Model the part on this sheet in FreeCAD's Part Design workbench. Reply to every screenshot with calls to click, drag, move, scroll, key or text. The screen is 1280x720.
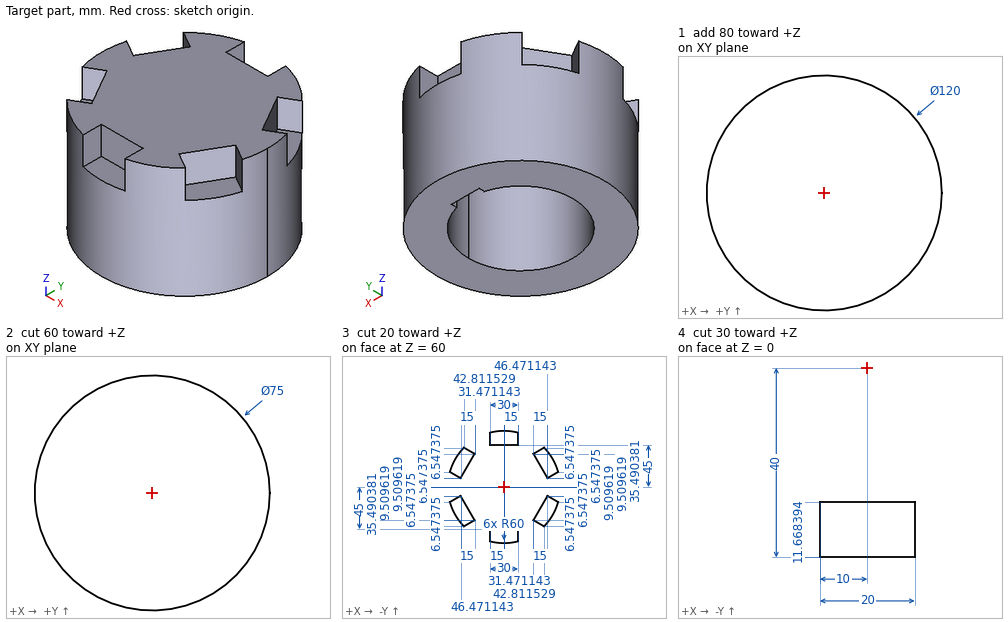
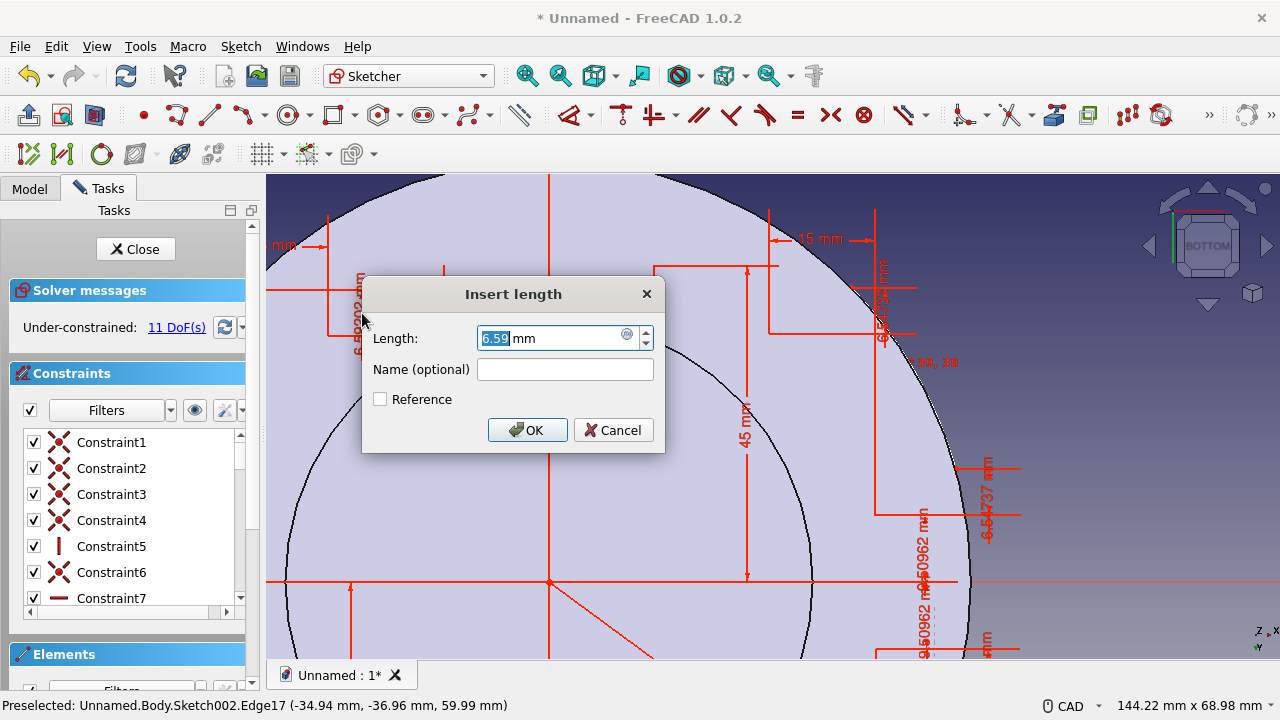
text(6.547375)
key(Return)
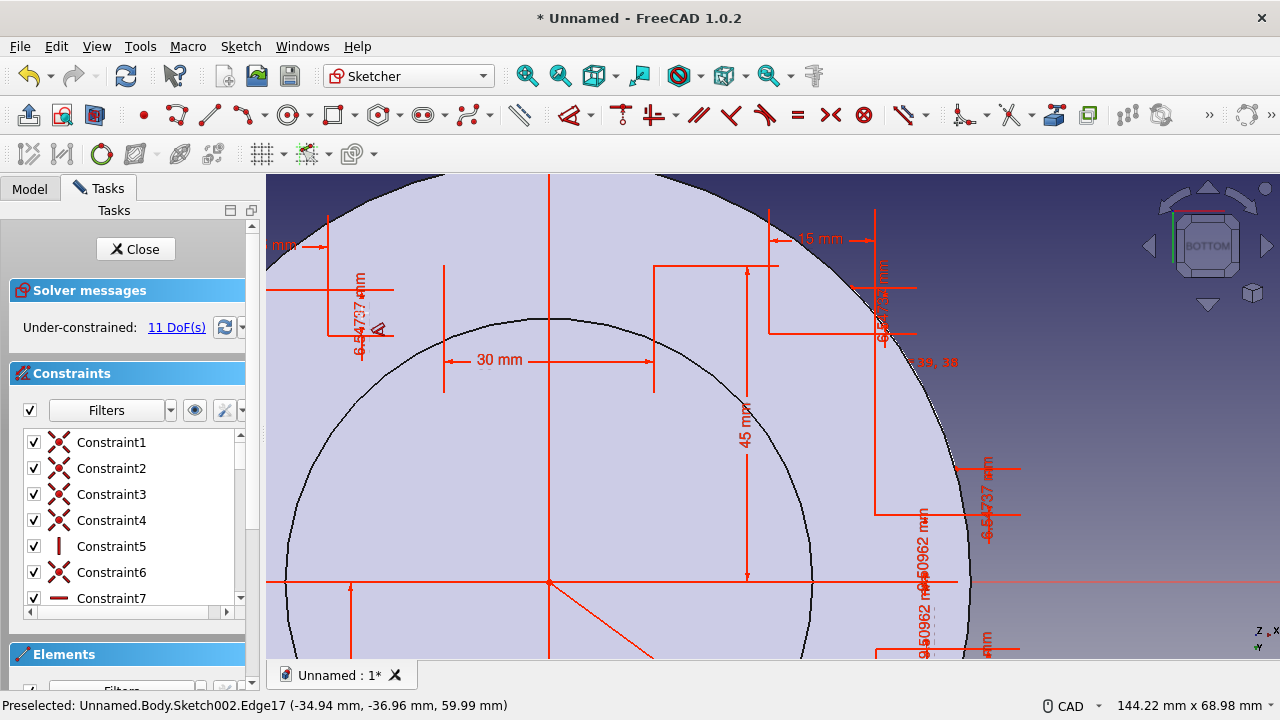
scroll(795, 320, down, 5)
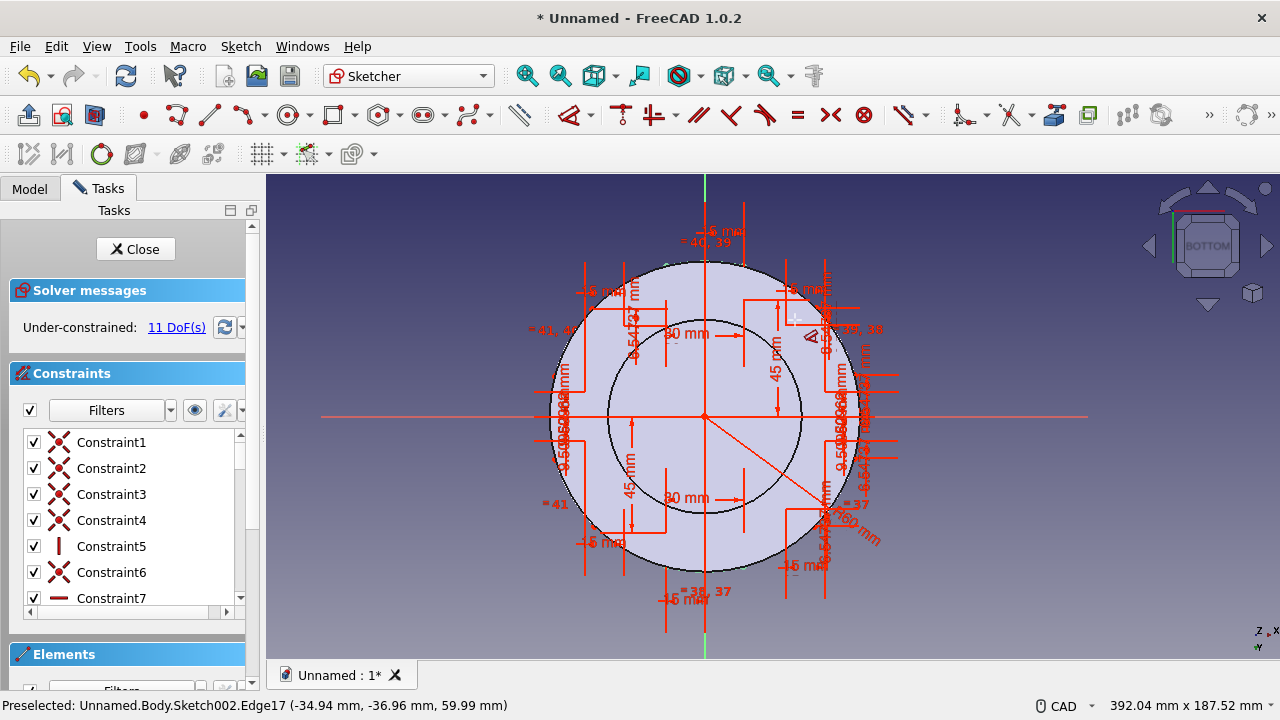
scroll(576, 387, up, 5)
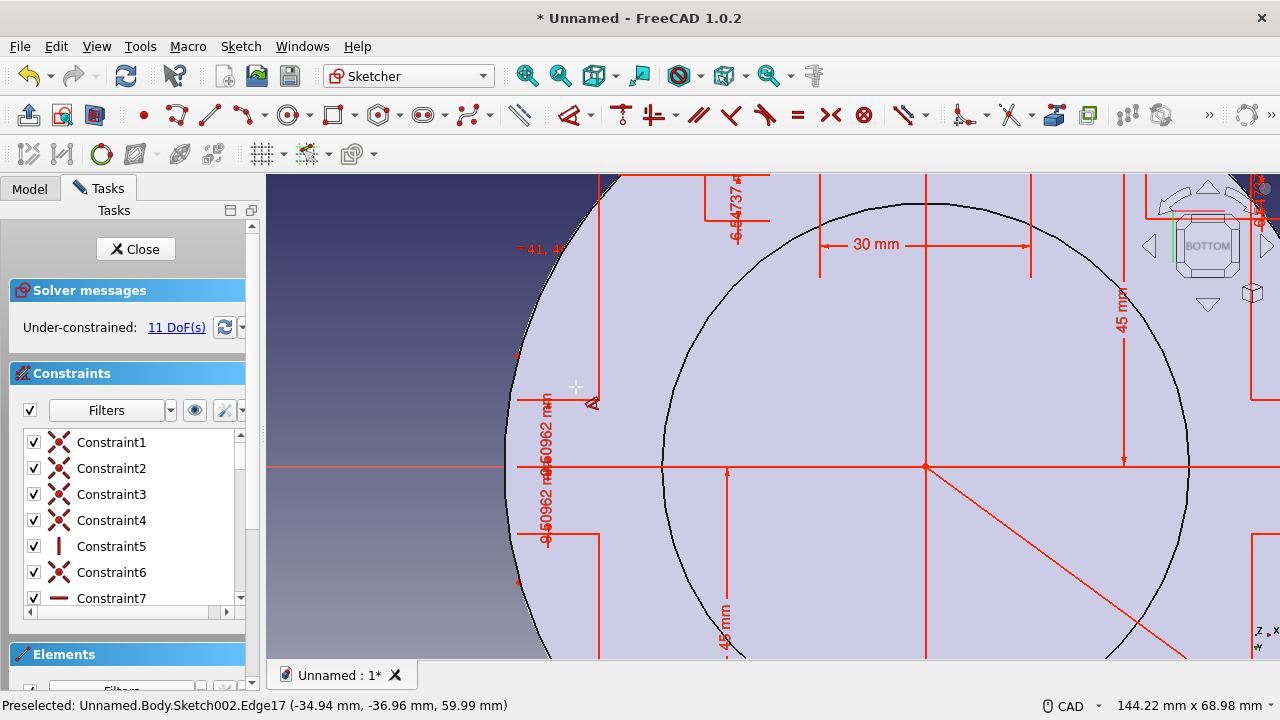
click(575, 387)
click(484, 378)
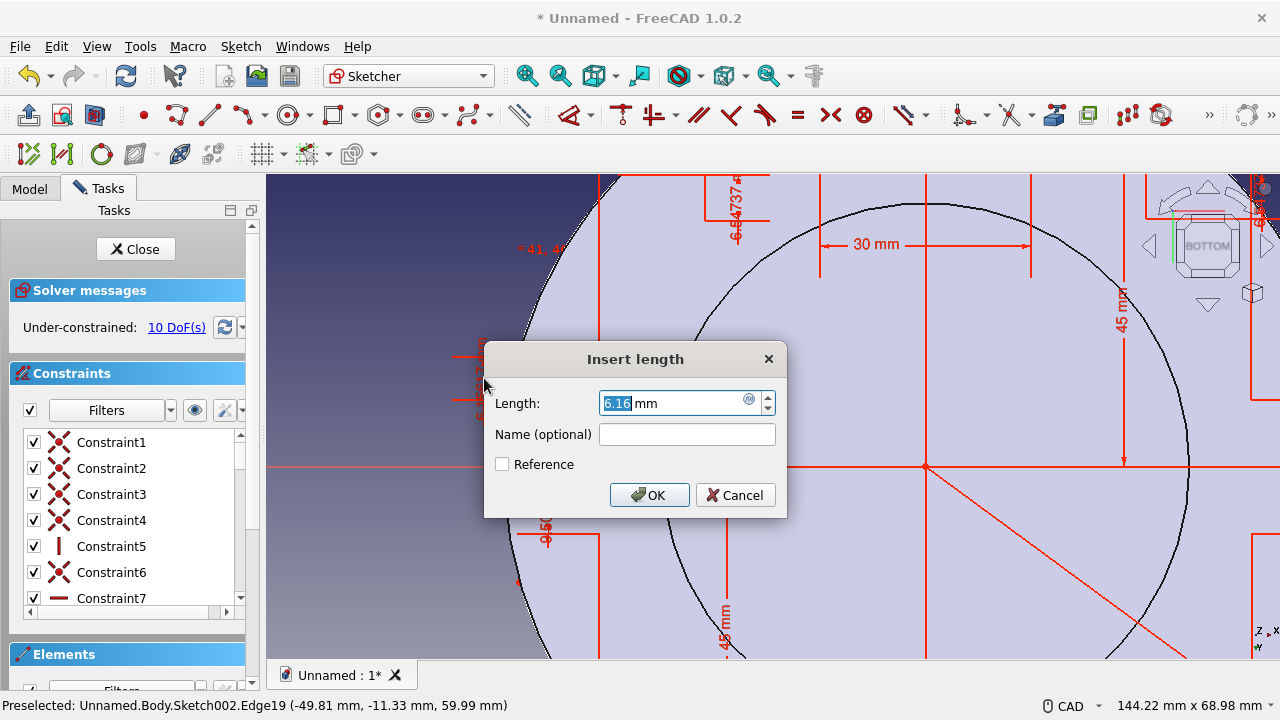
text(6.547375)
key(Return)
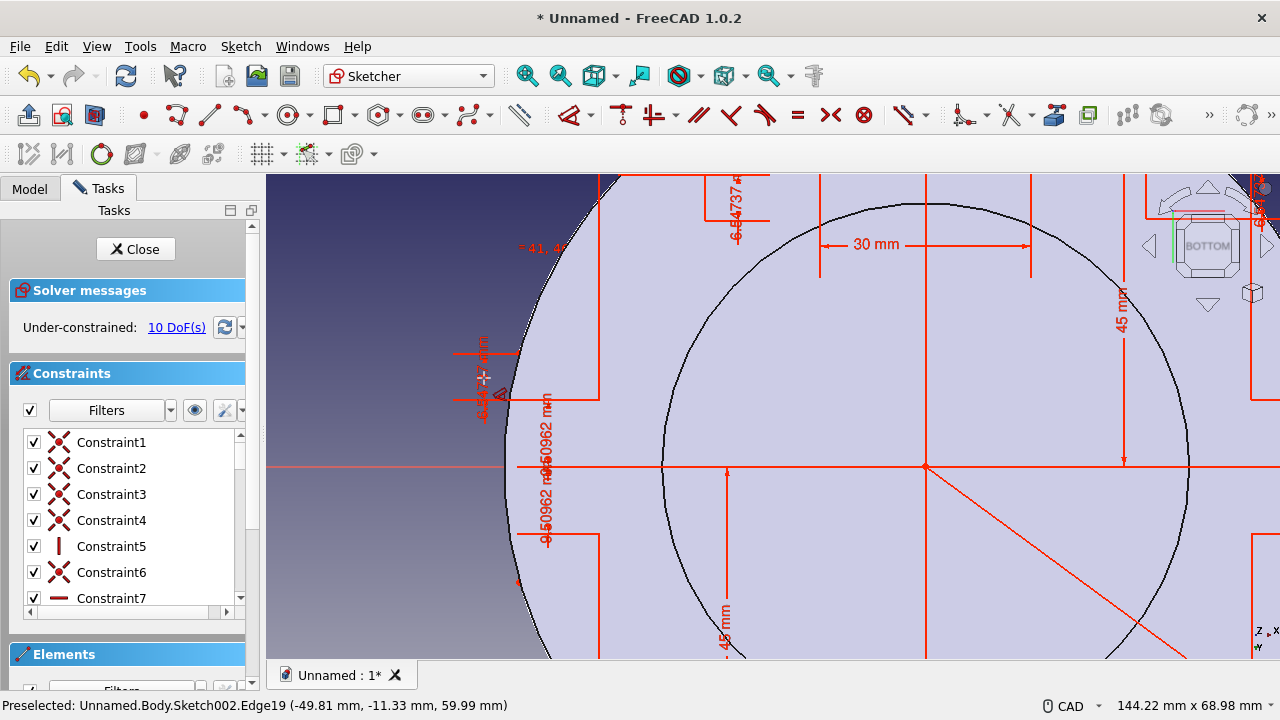
click(544, 568)
click(486, 558)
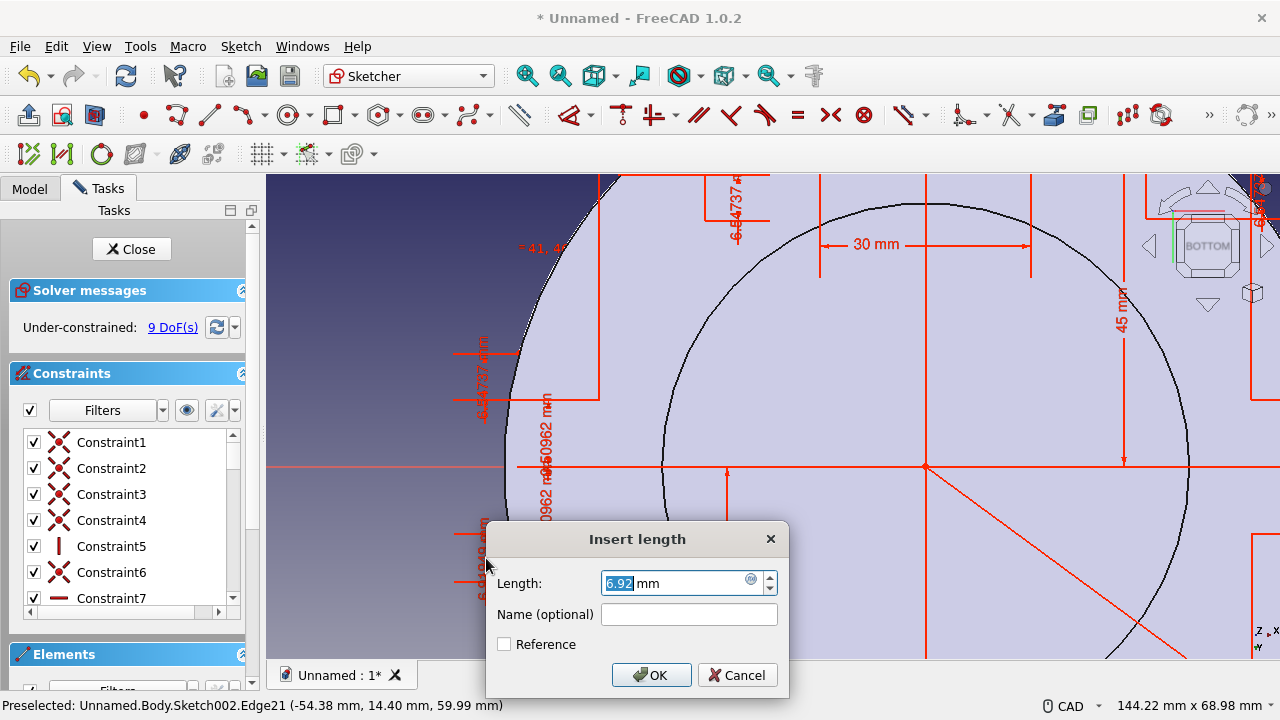
text(6.547375)
key(Return)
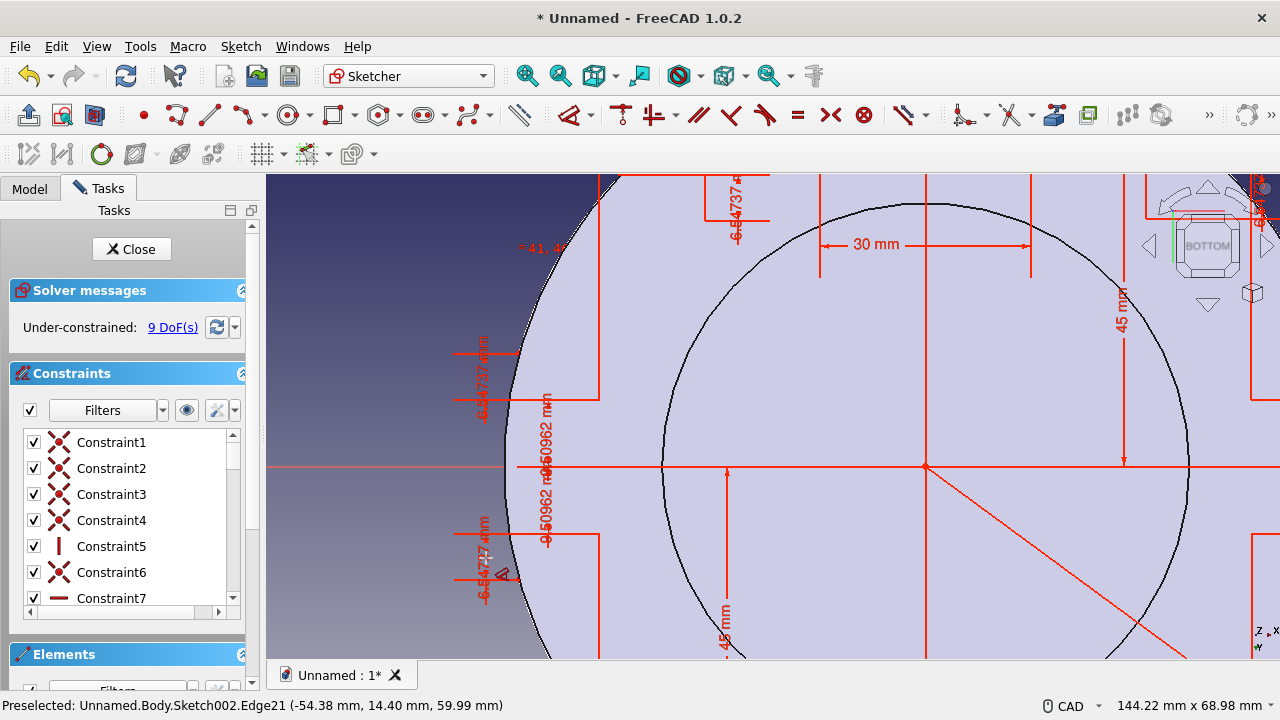
scroll(576, 387, down, 5)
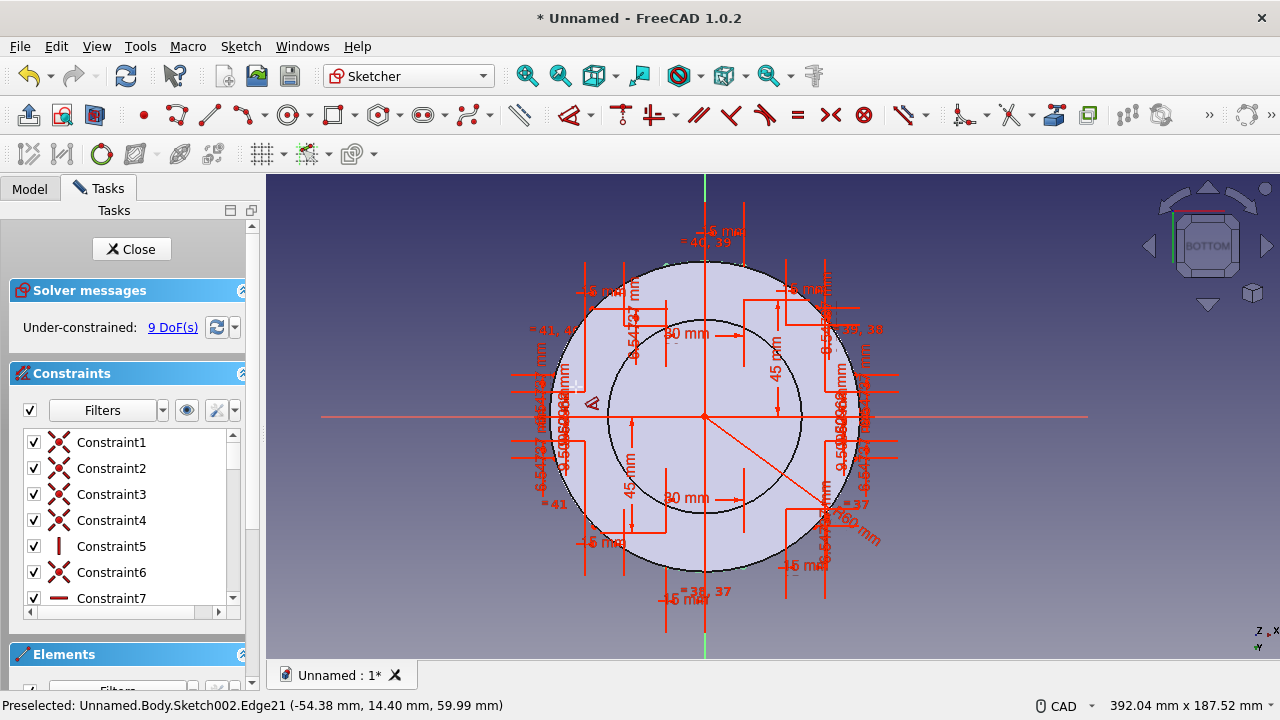
scroll(615, 514, up, 5)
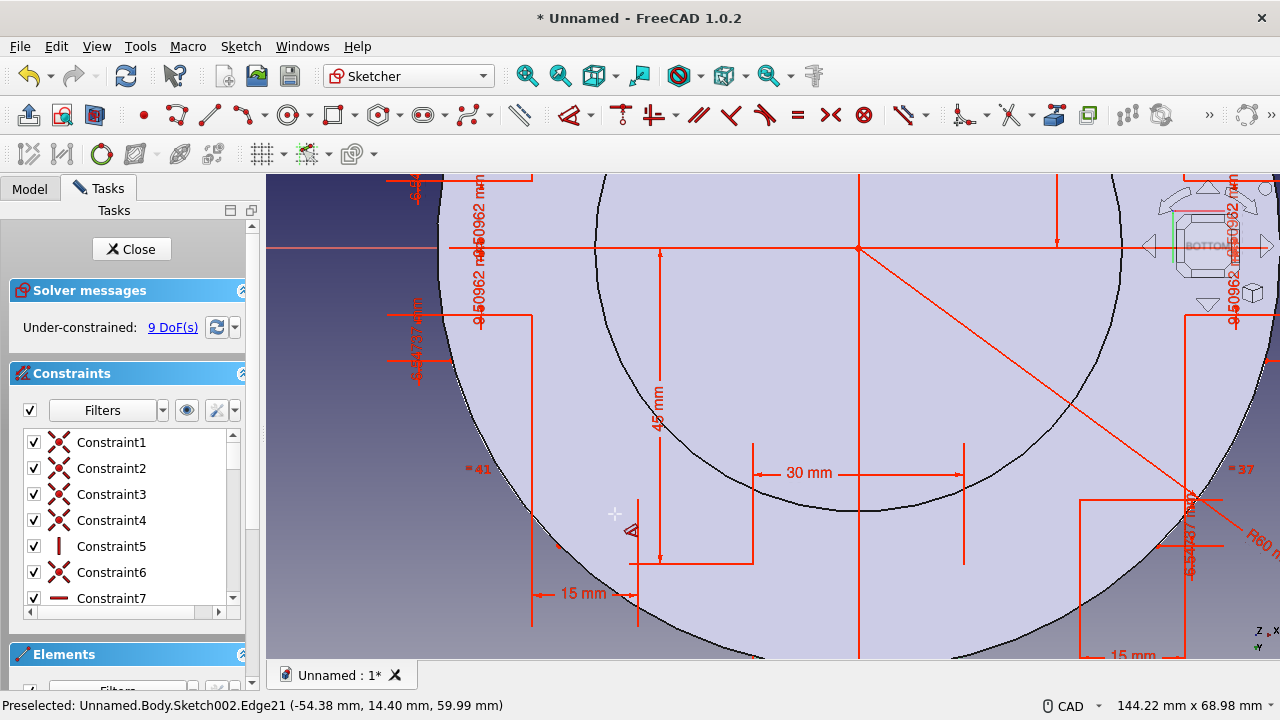
click(614, 513)
click(526, 533)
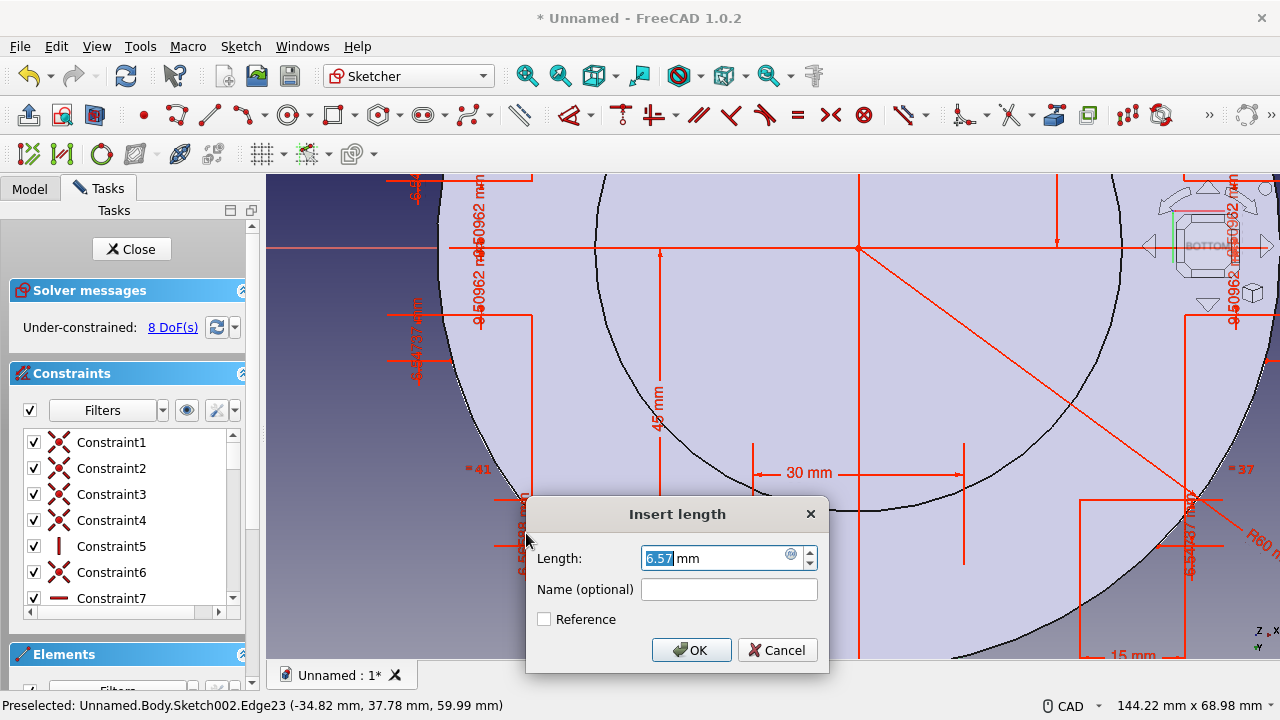
text(6.547375)
key(Return)